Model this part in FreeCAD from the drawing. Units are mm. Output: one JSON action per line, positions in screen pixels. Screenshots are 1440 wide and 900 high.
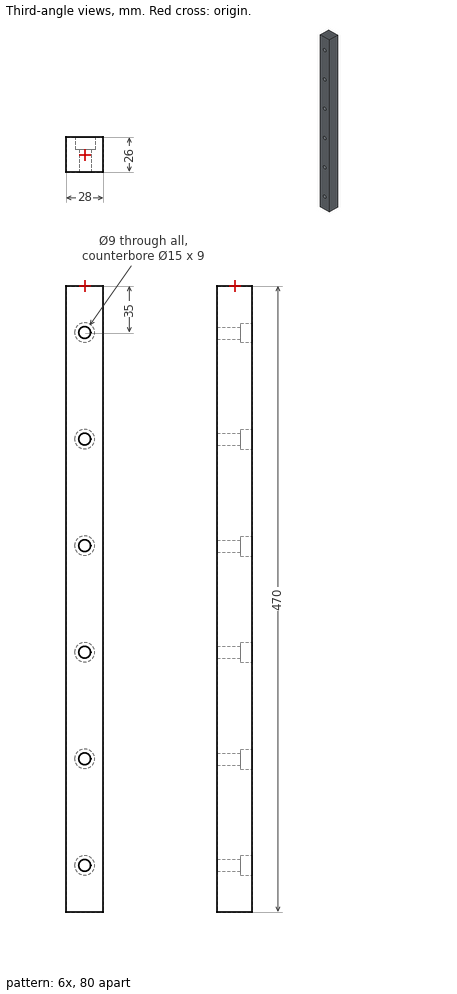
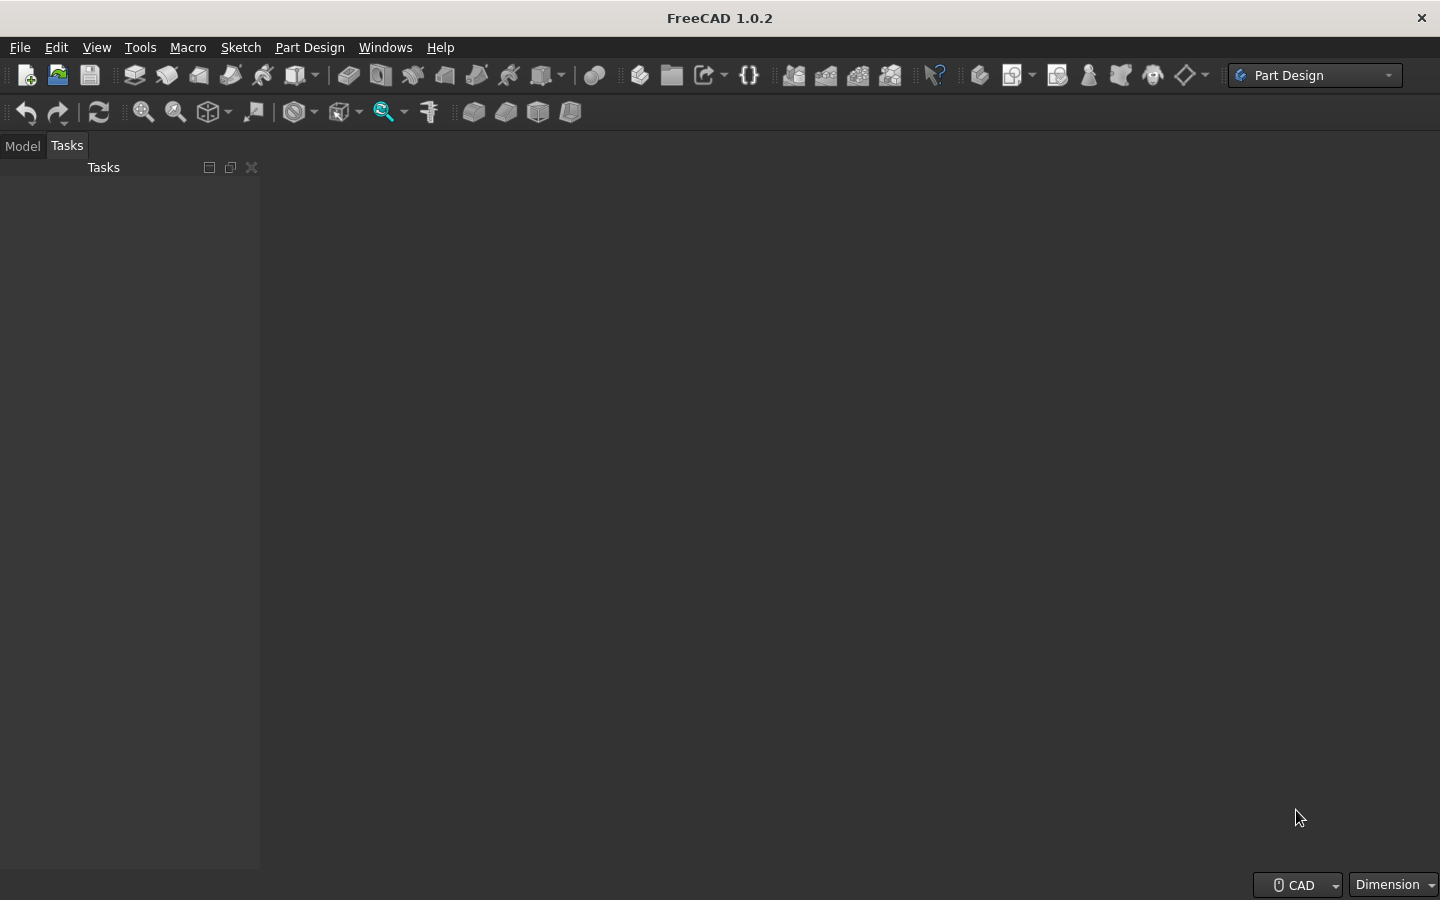
{"action": "left_click", "coordinate": [26, 76]}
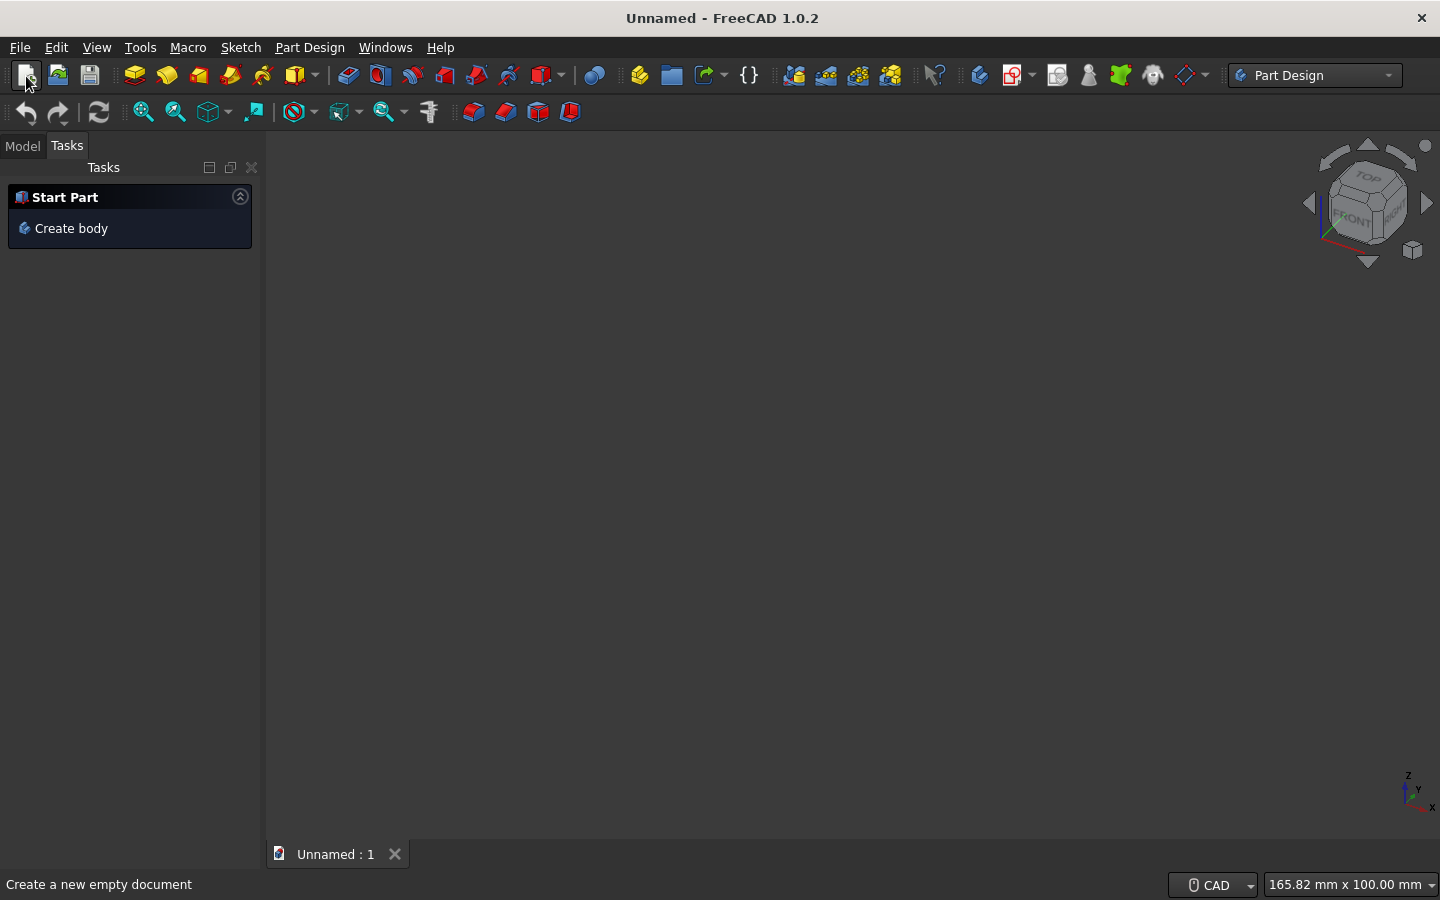
{"action": "left_click", "coordinate": [1012, 76]}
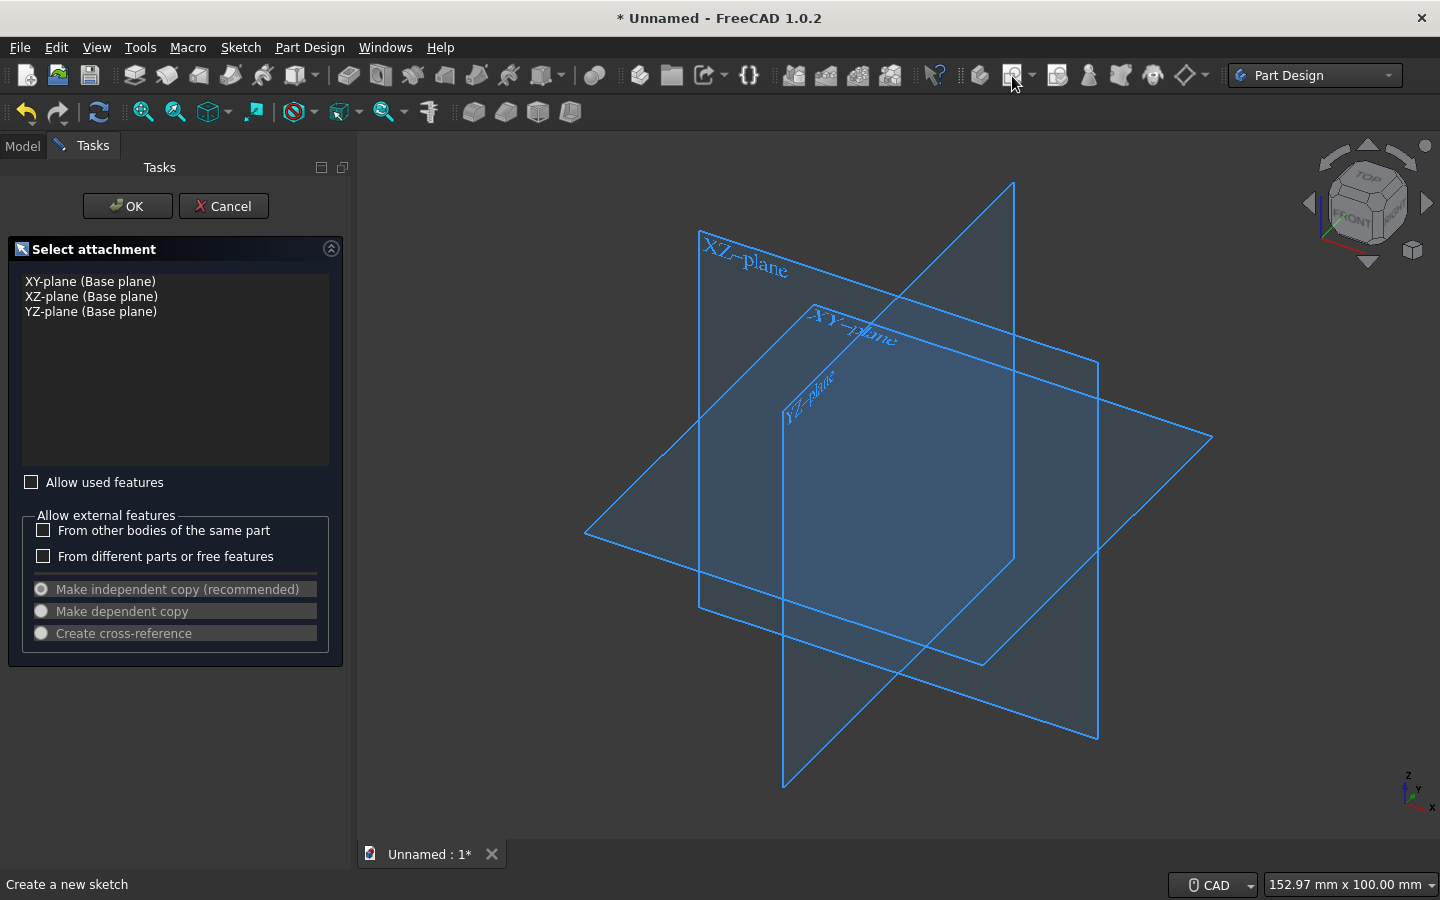
{"action": "left_click", "coordinate": [82, 282]}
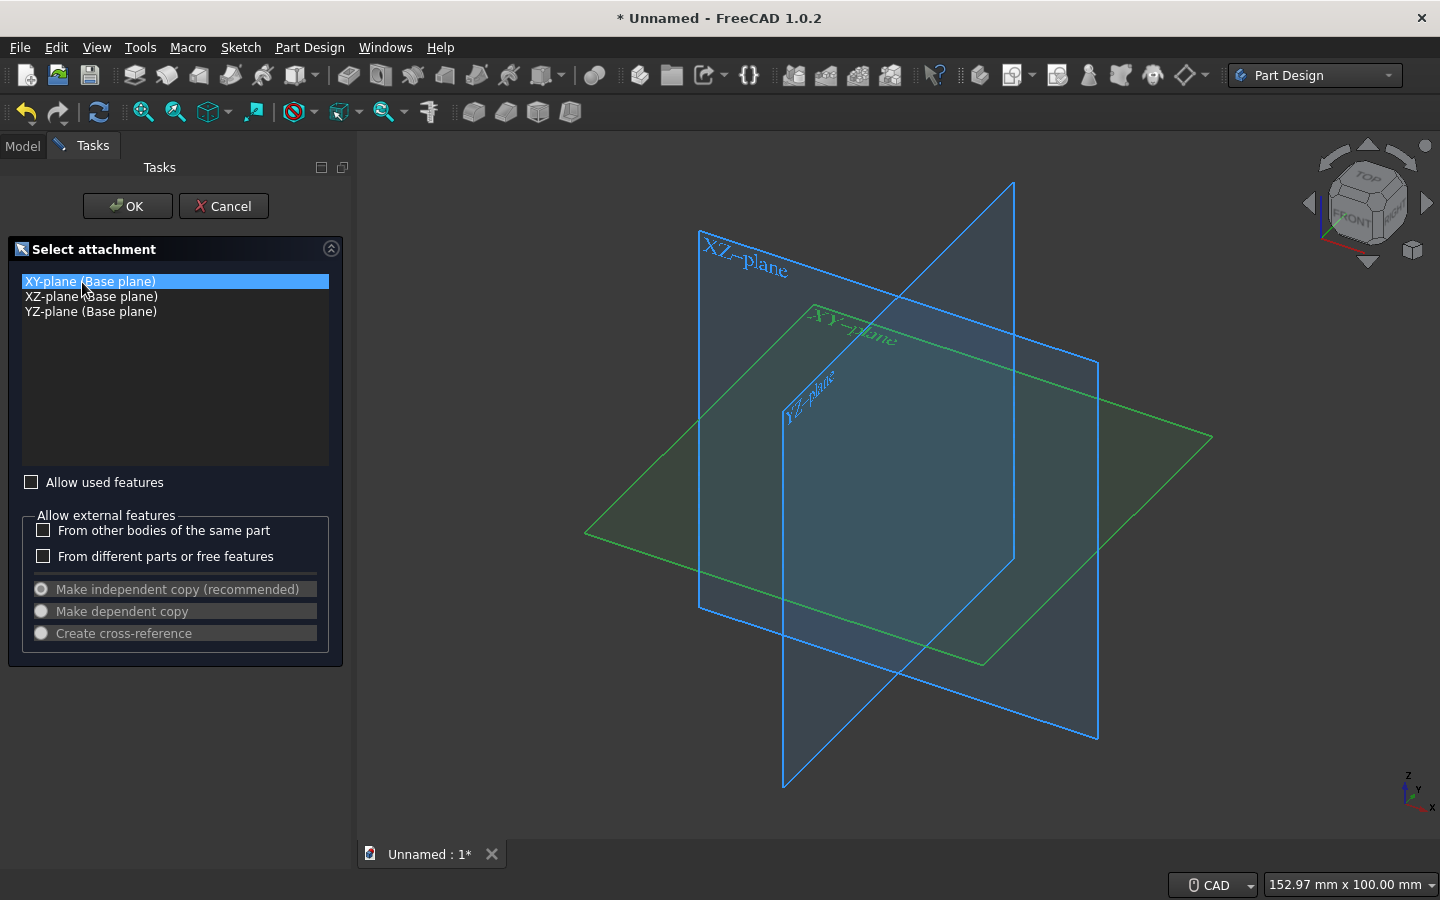
{"action": "left_click", "coordinate": [128, 206]}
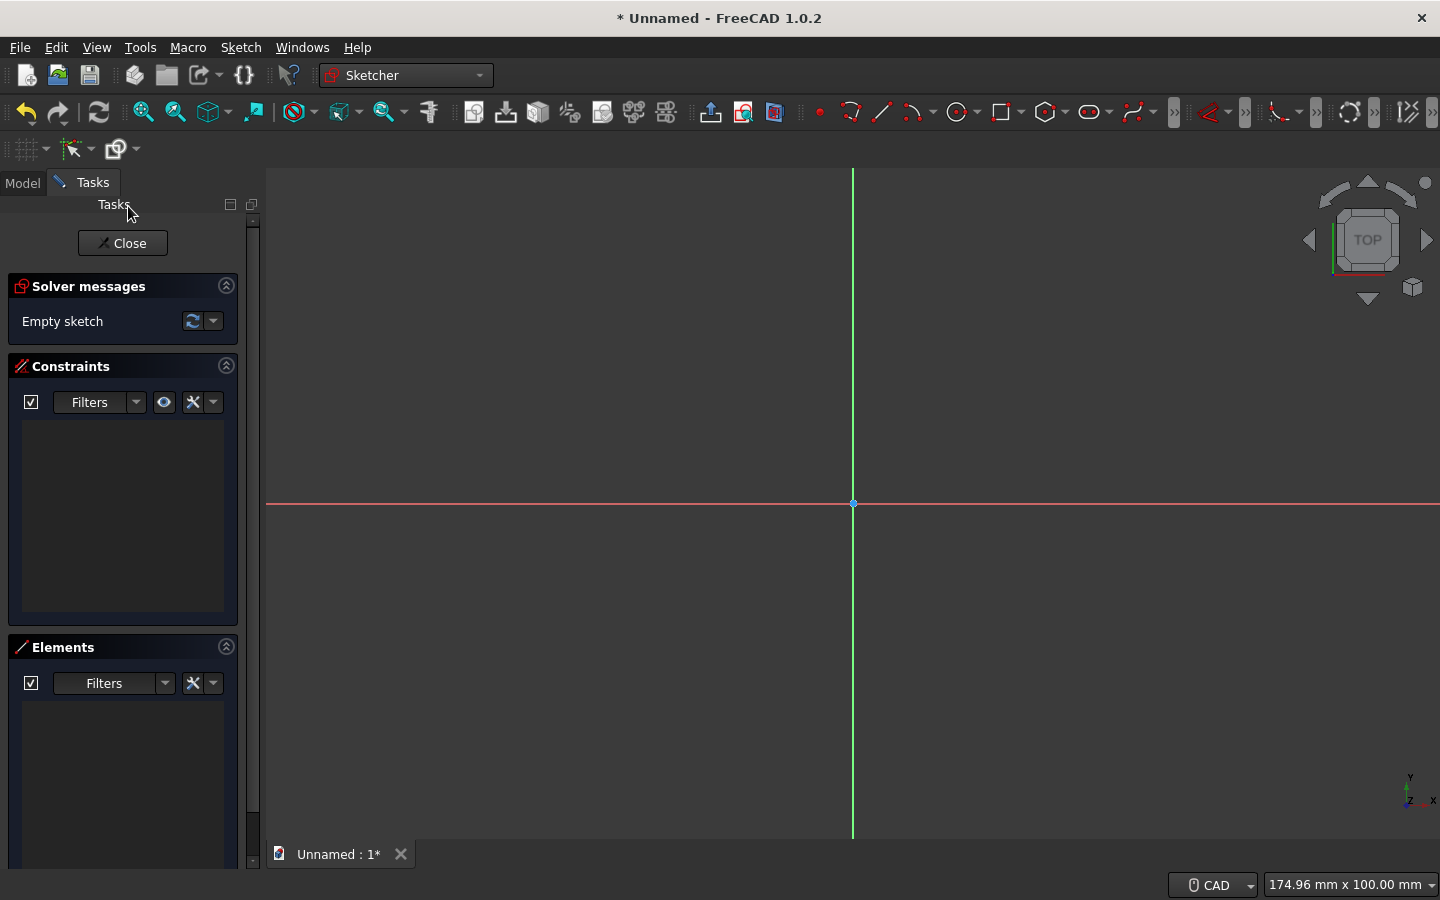
{"action": "scroll", "coordinate": [893, 504], "scroll_direction": "up", "scroll_amount": 5}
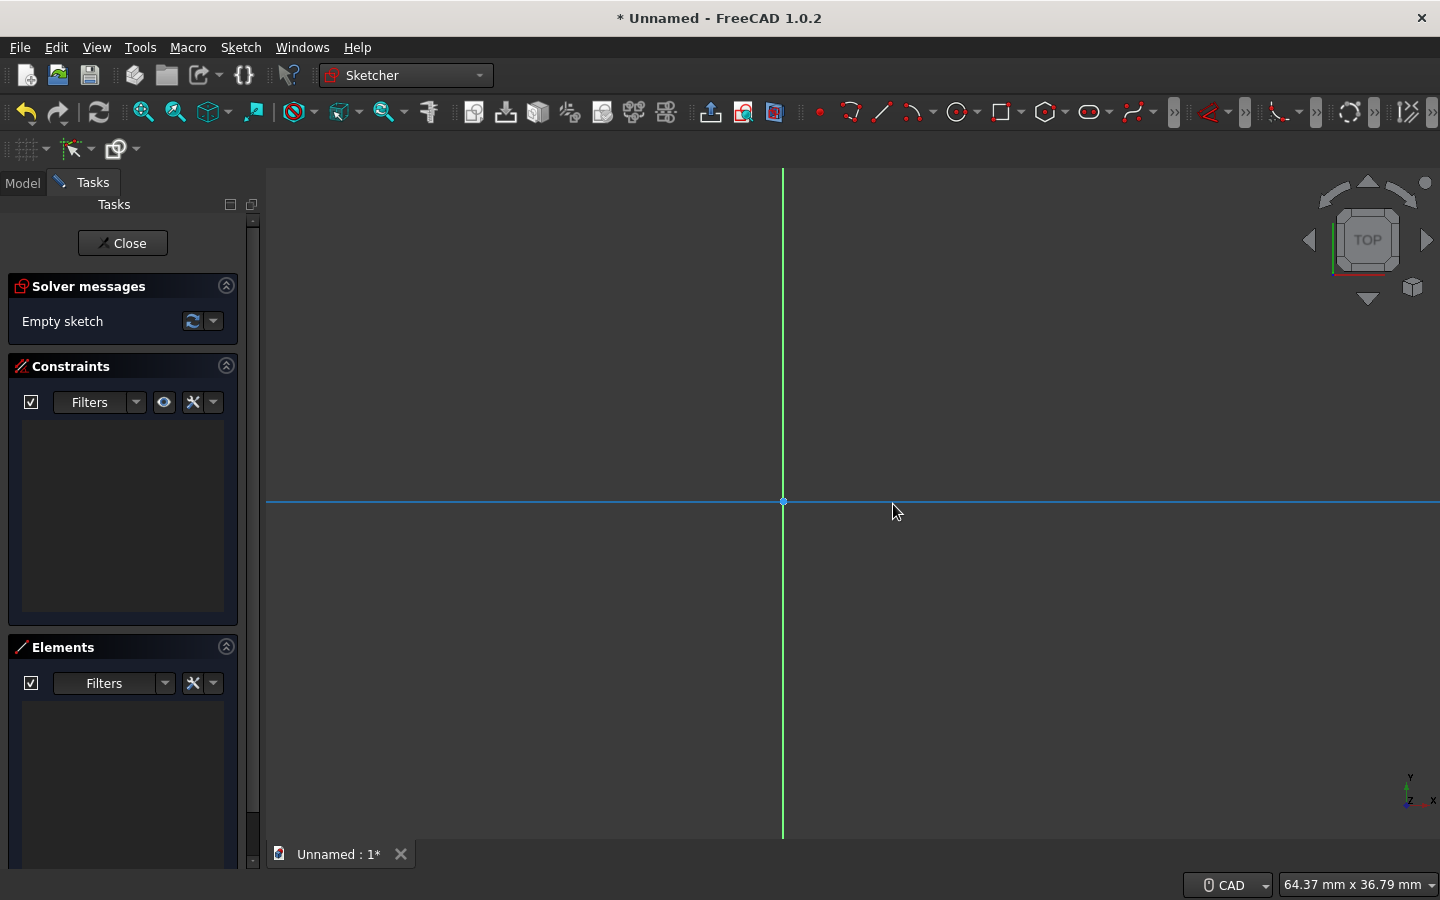
{"action": "left_click", "coordinate": [1024, 112]}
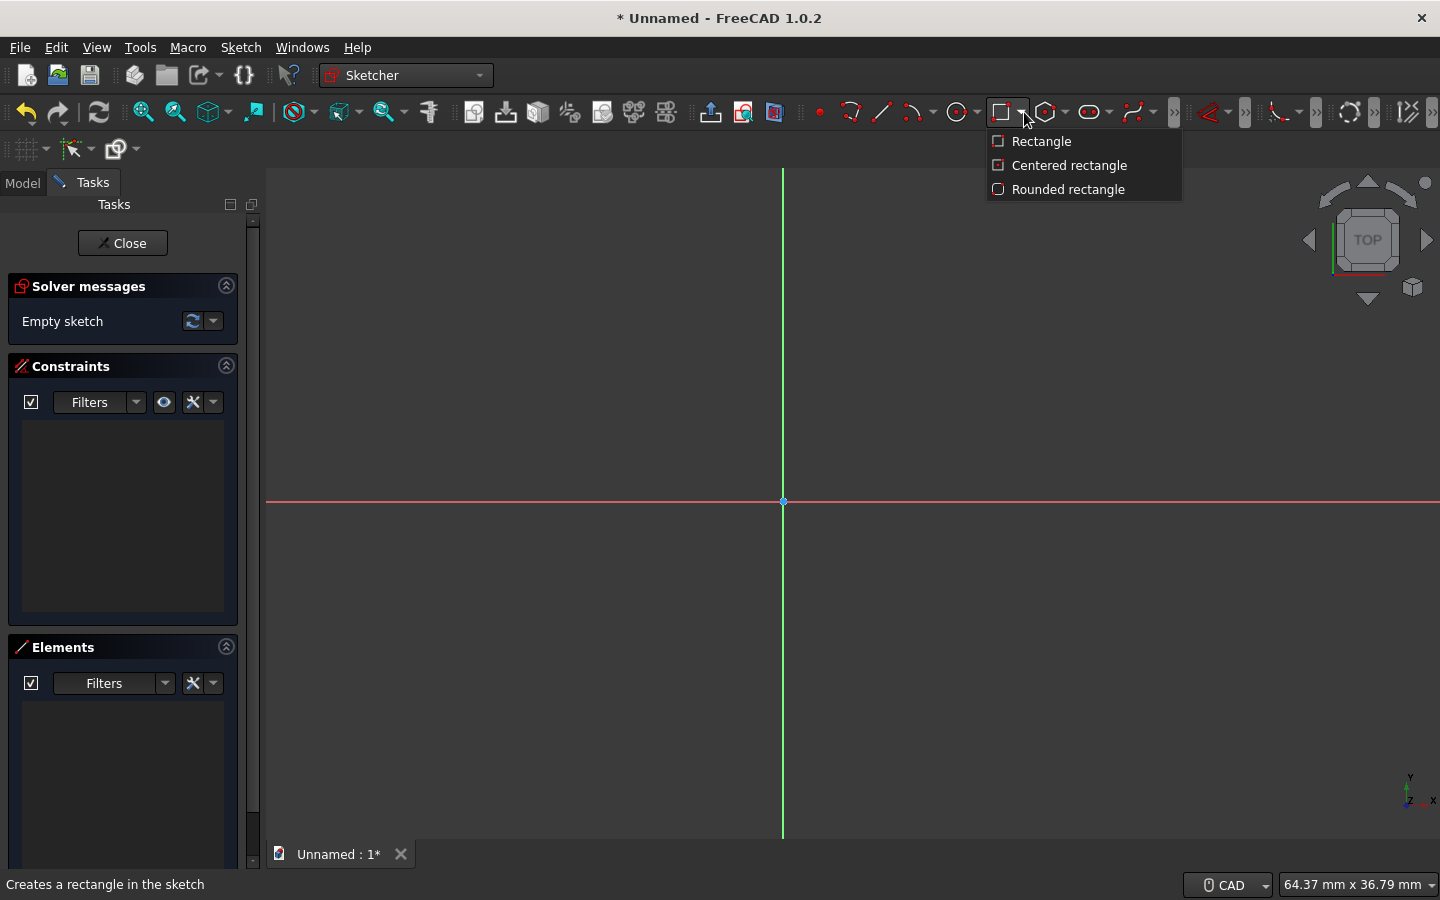
{"action": "left_click", "coordinate": [1084, 165]}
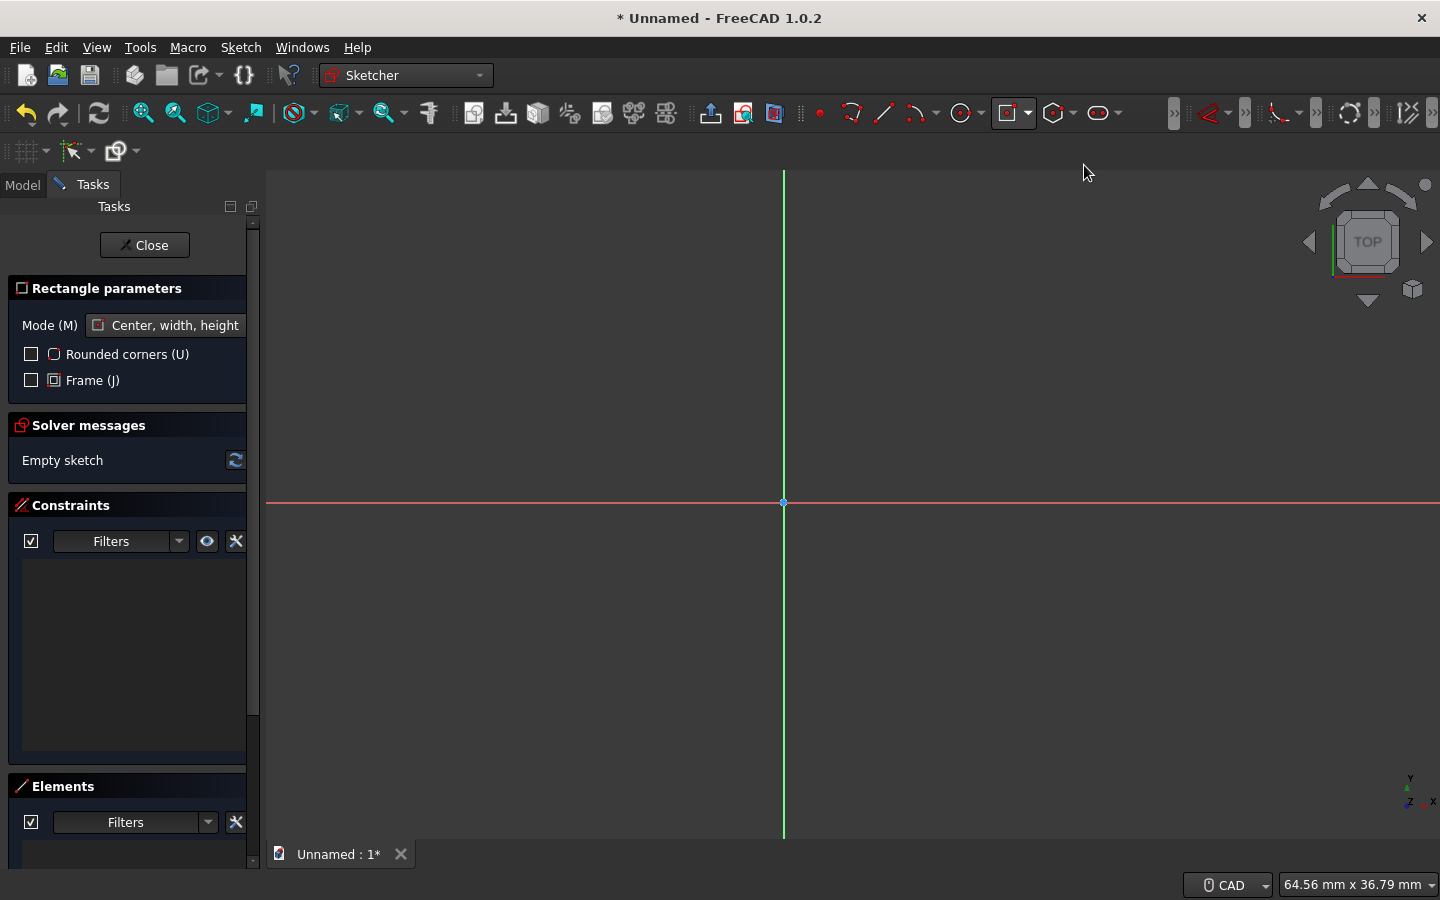
{"action": "left_click", "coordinate": [784, 503]}
{"action": "mouse_move", "coordinate": [1038, 266]}